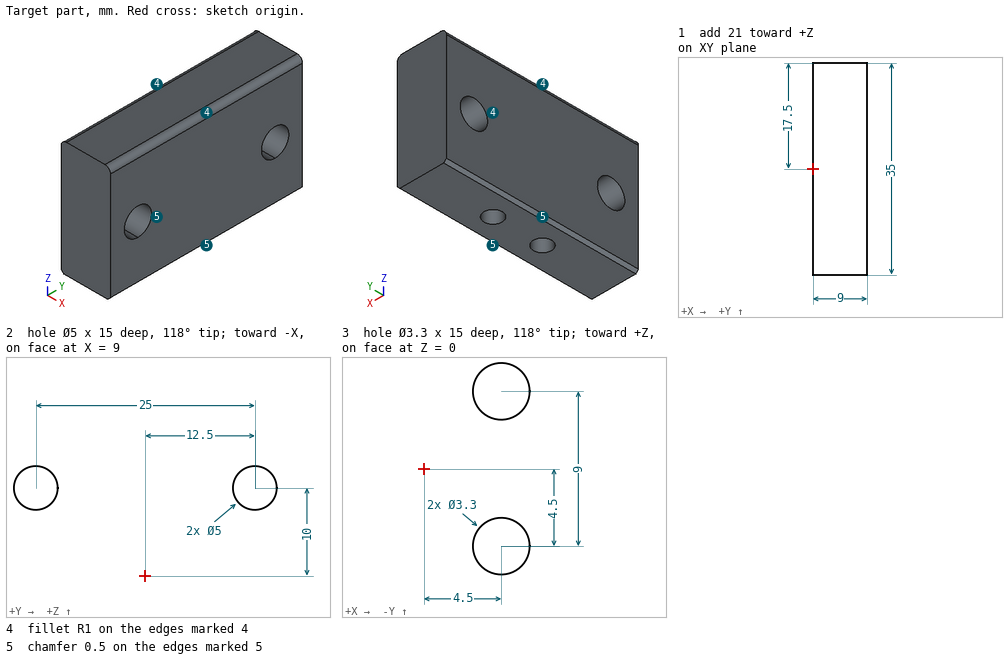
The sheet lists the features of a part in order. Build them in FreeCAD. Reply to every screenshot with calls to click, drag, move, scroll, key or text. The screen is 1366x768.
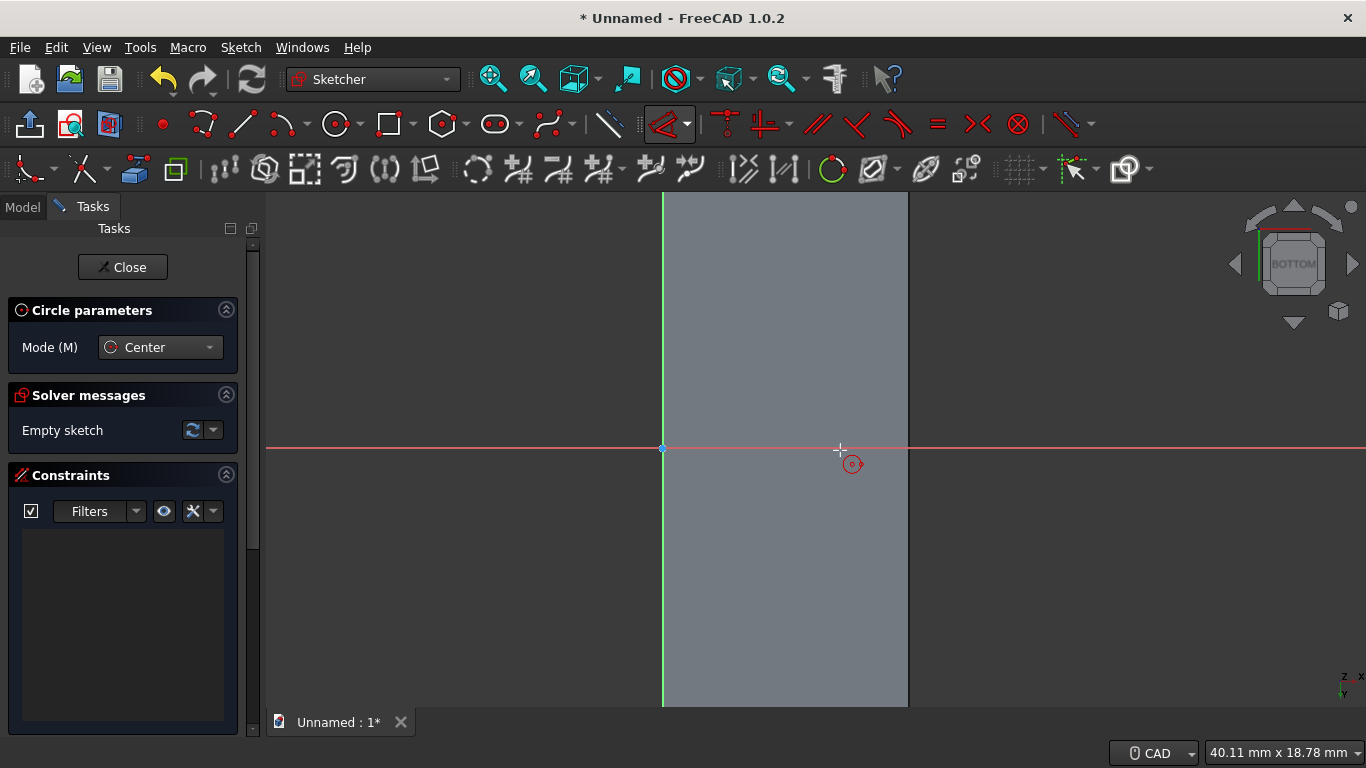
click(786, 572)
move(818, 540)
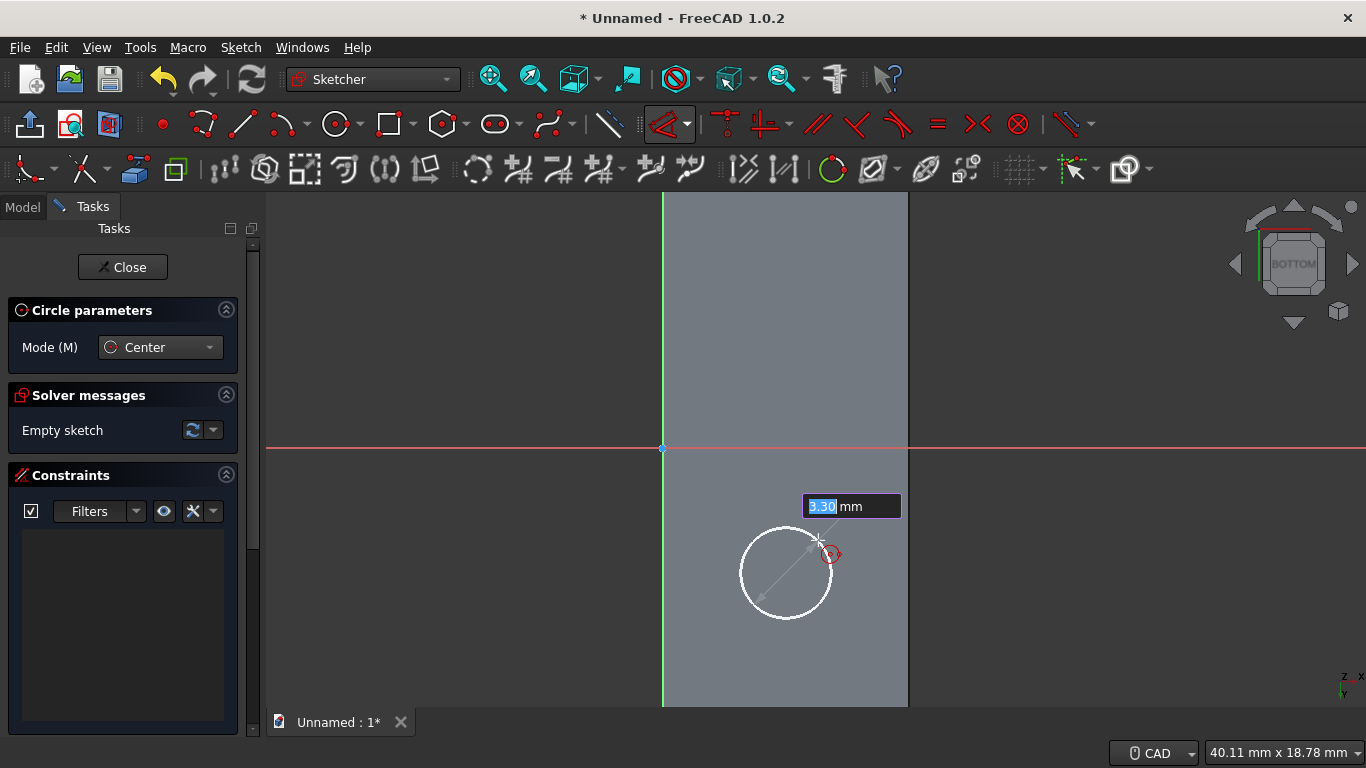
text(3.3)
key(Return)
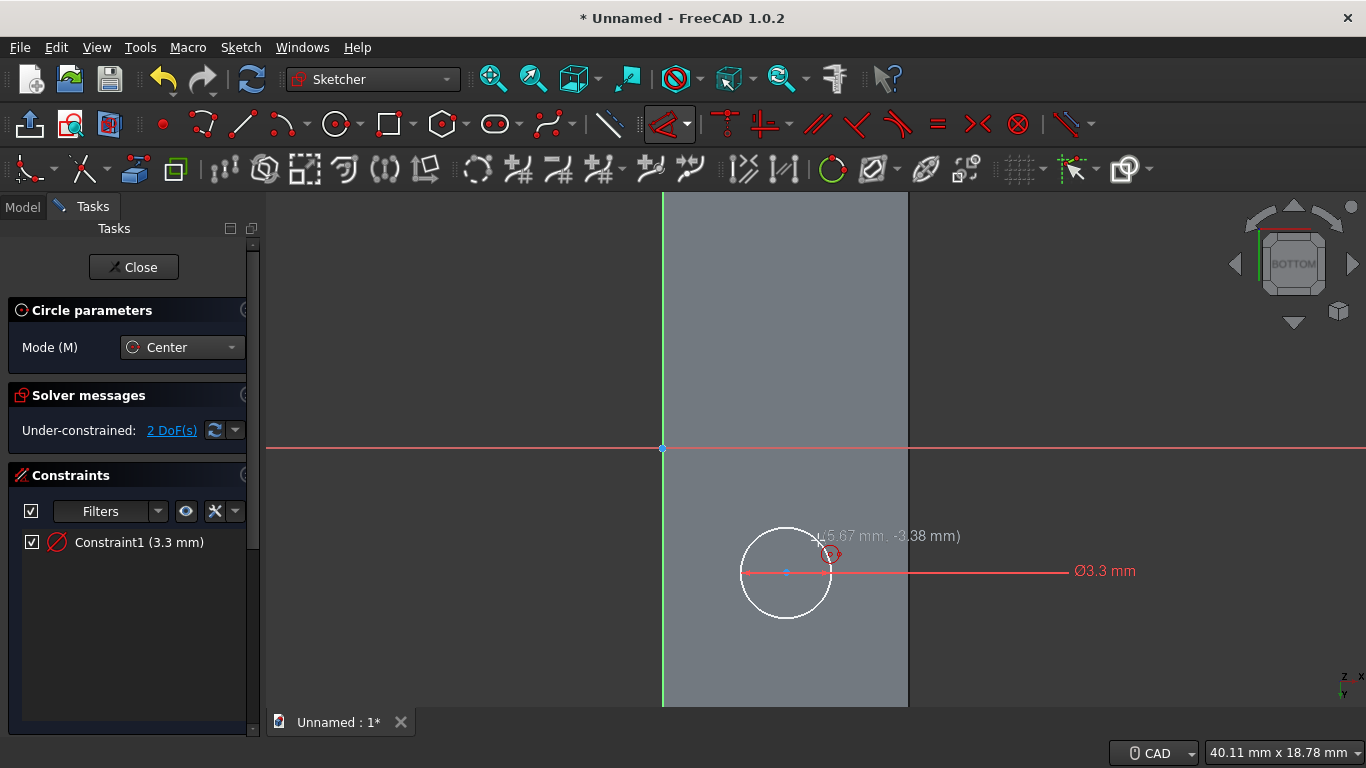
click(786, 325)
move(818, 293)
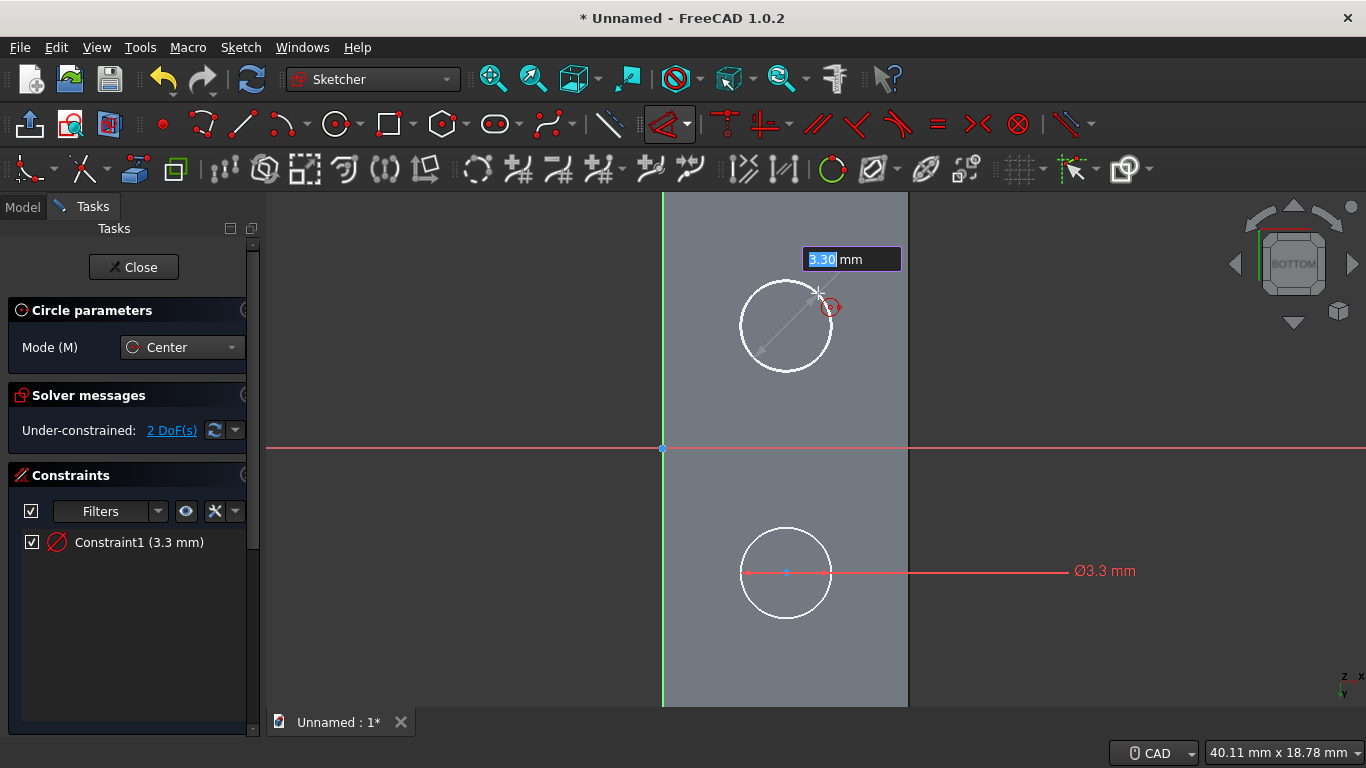
text(3.3)
key(Return)
key(Escape)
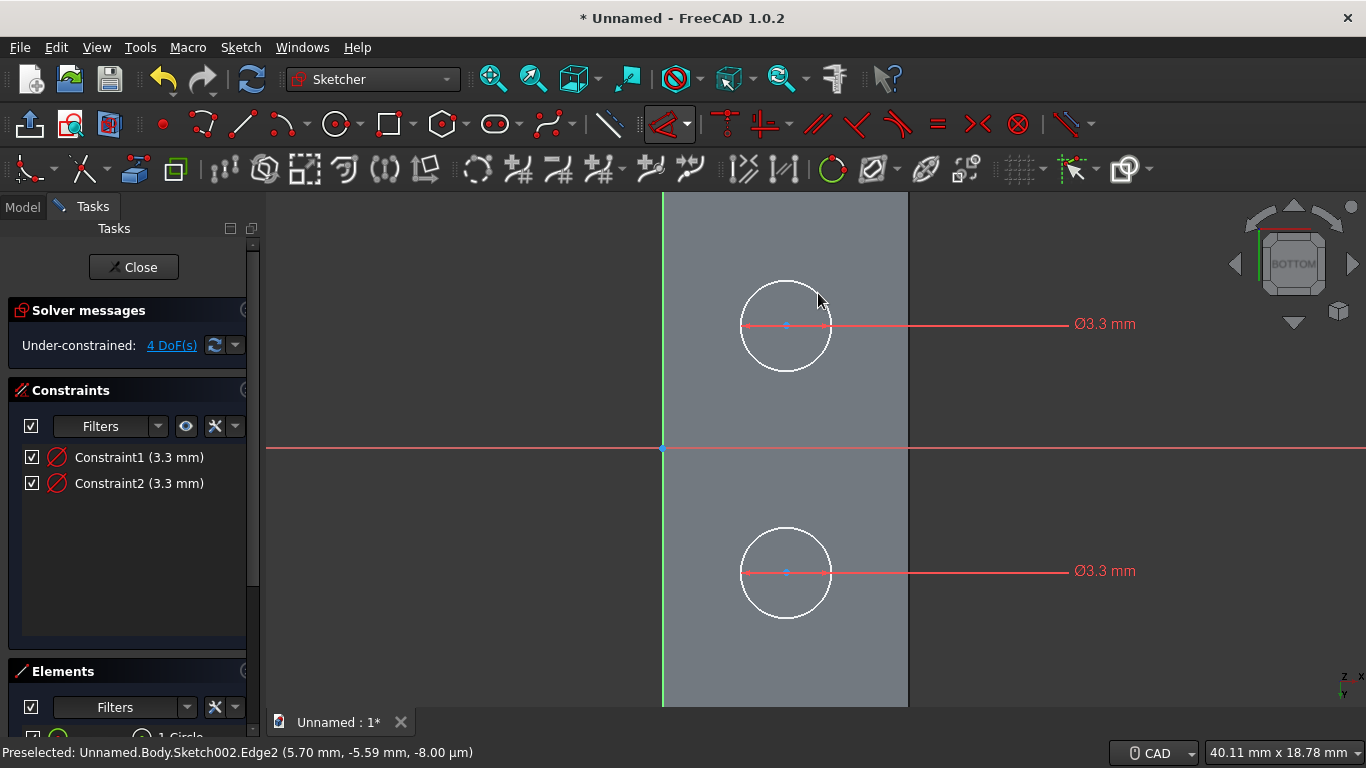
click(786, 573)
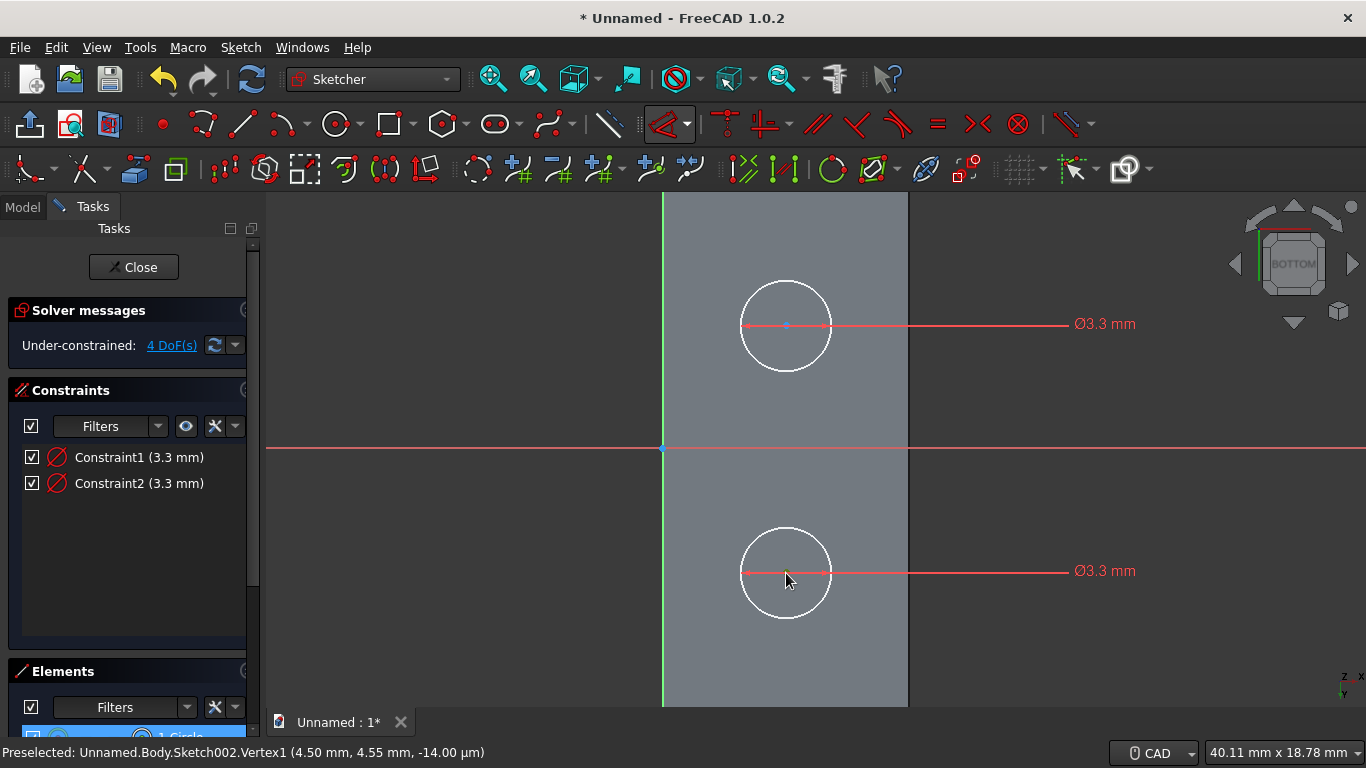
click(786, 326)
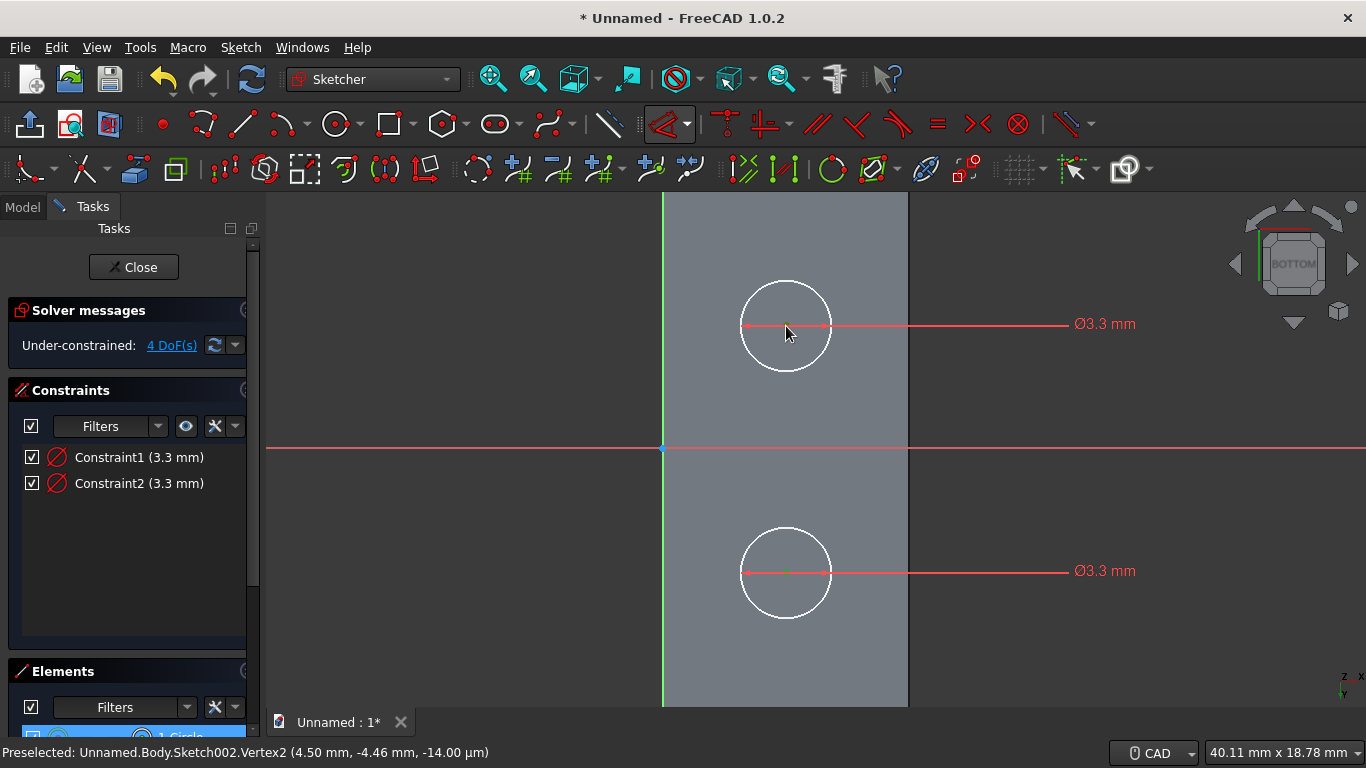
key(v)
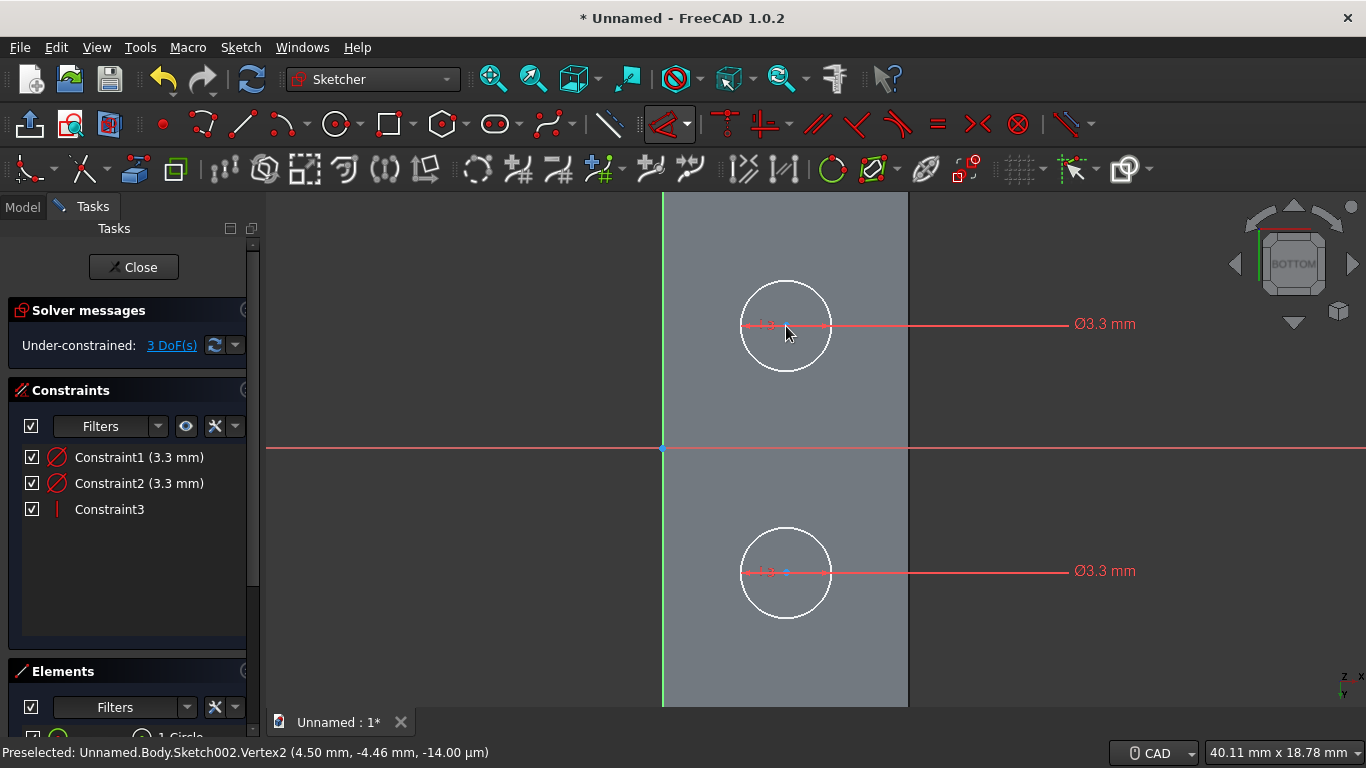
click(786, 573)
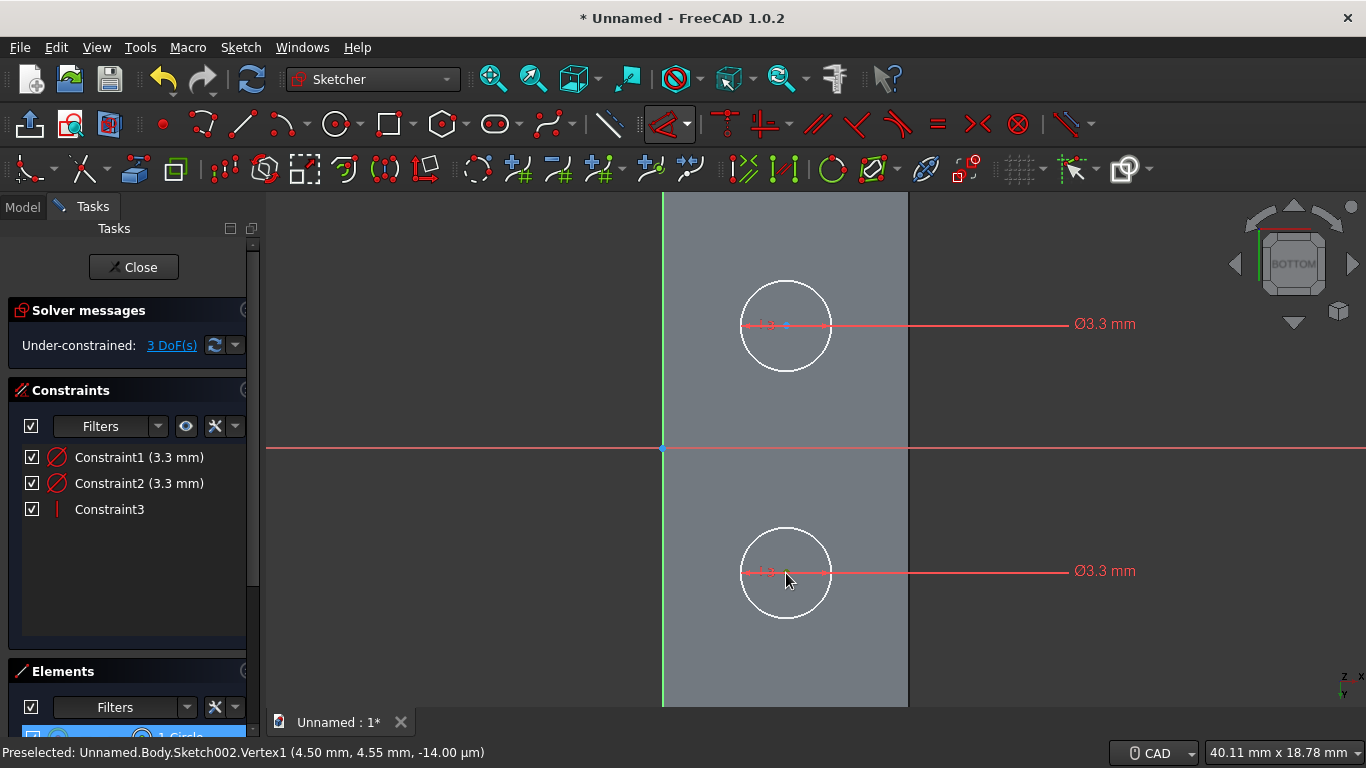
click(786, 326)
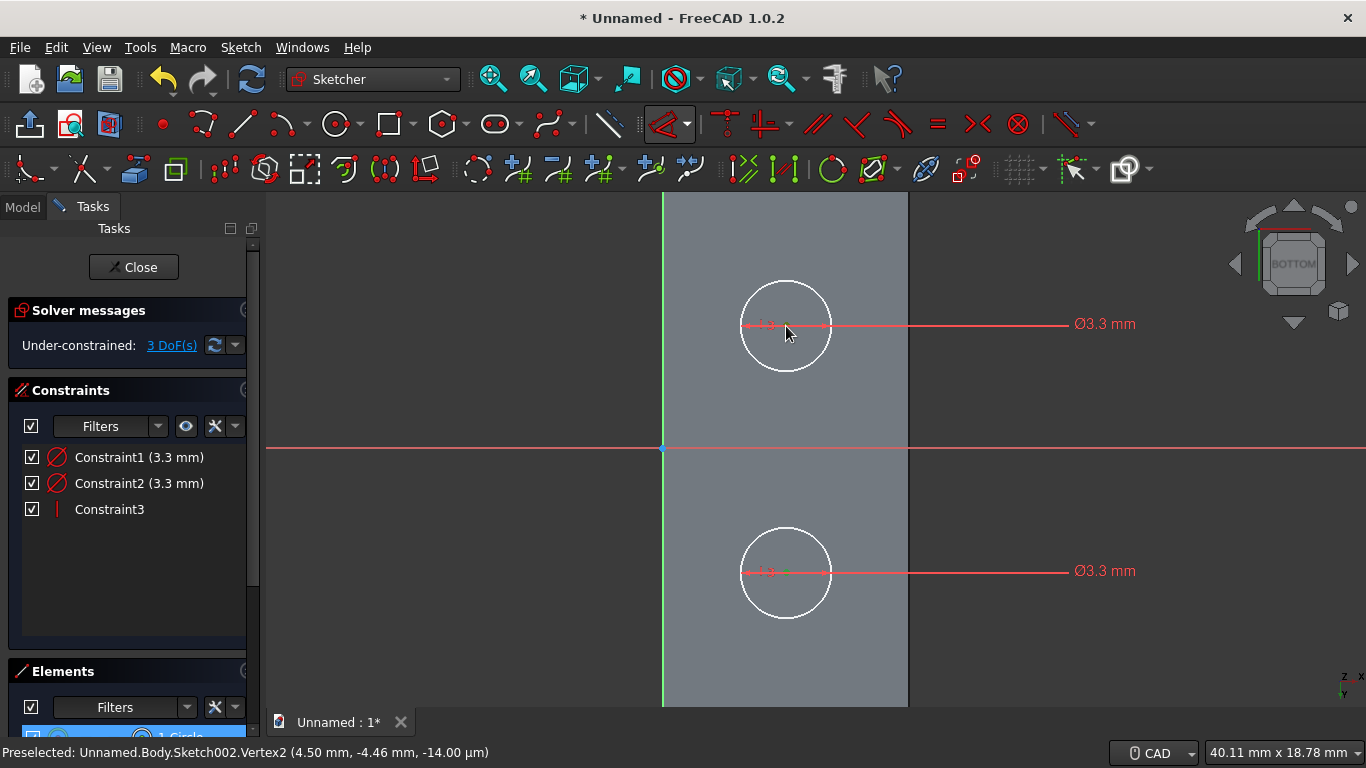
key(i)